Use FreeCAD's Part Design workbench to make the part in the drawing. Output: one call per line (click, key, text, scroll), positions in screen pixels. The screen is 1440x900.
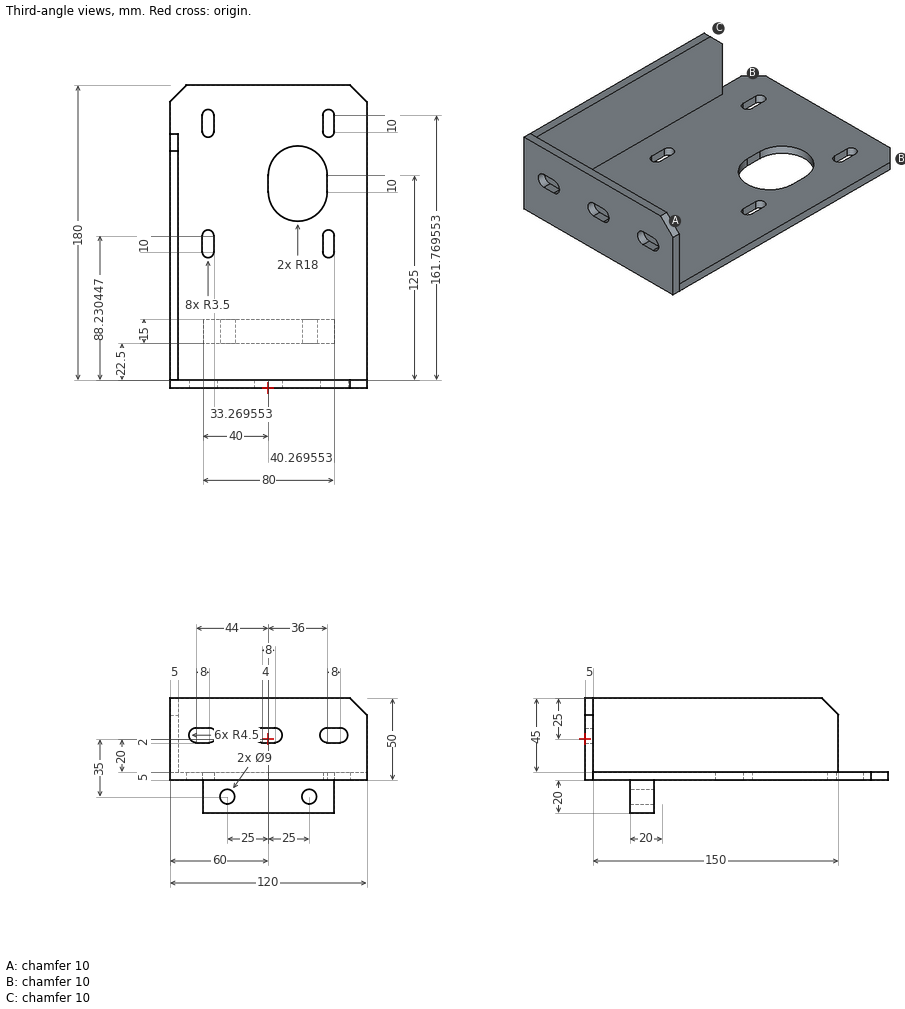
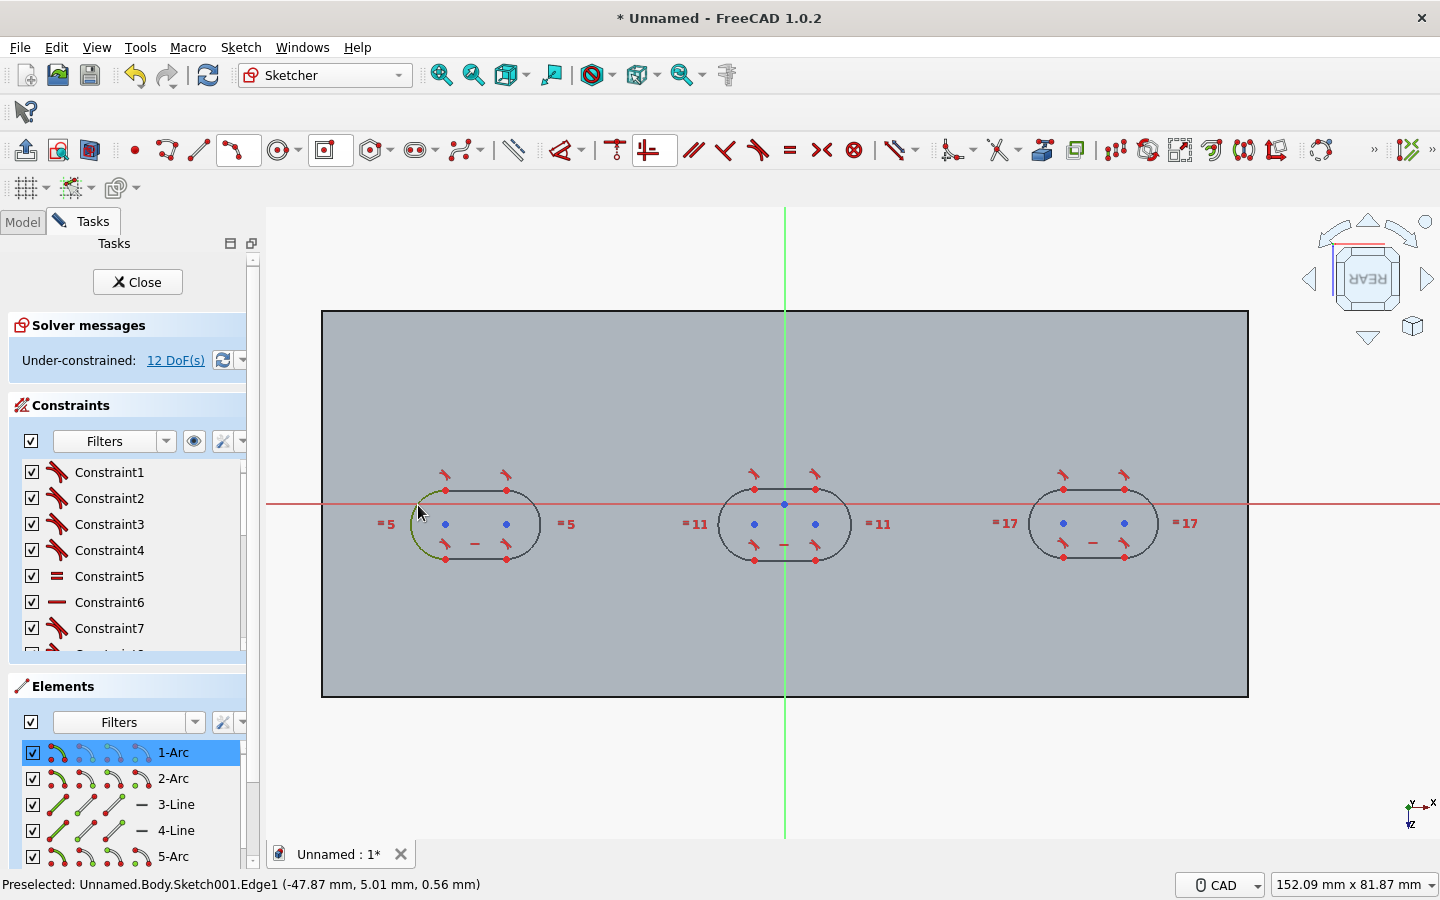
click(725, 504)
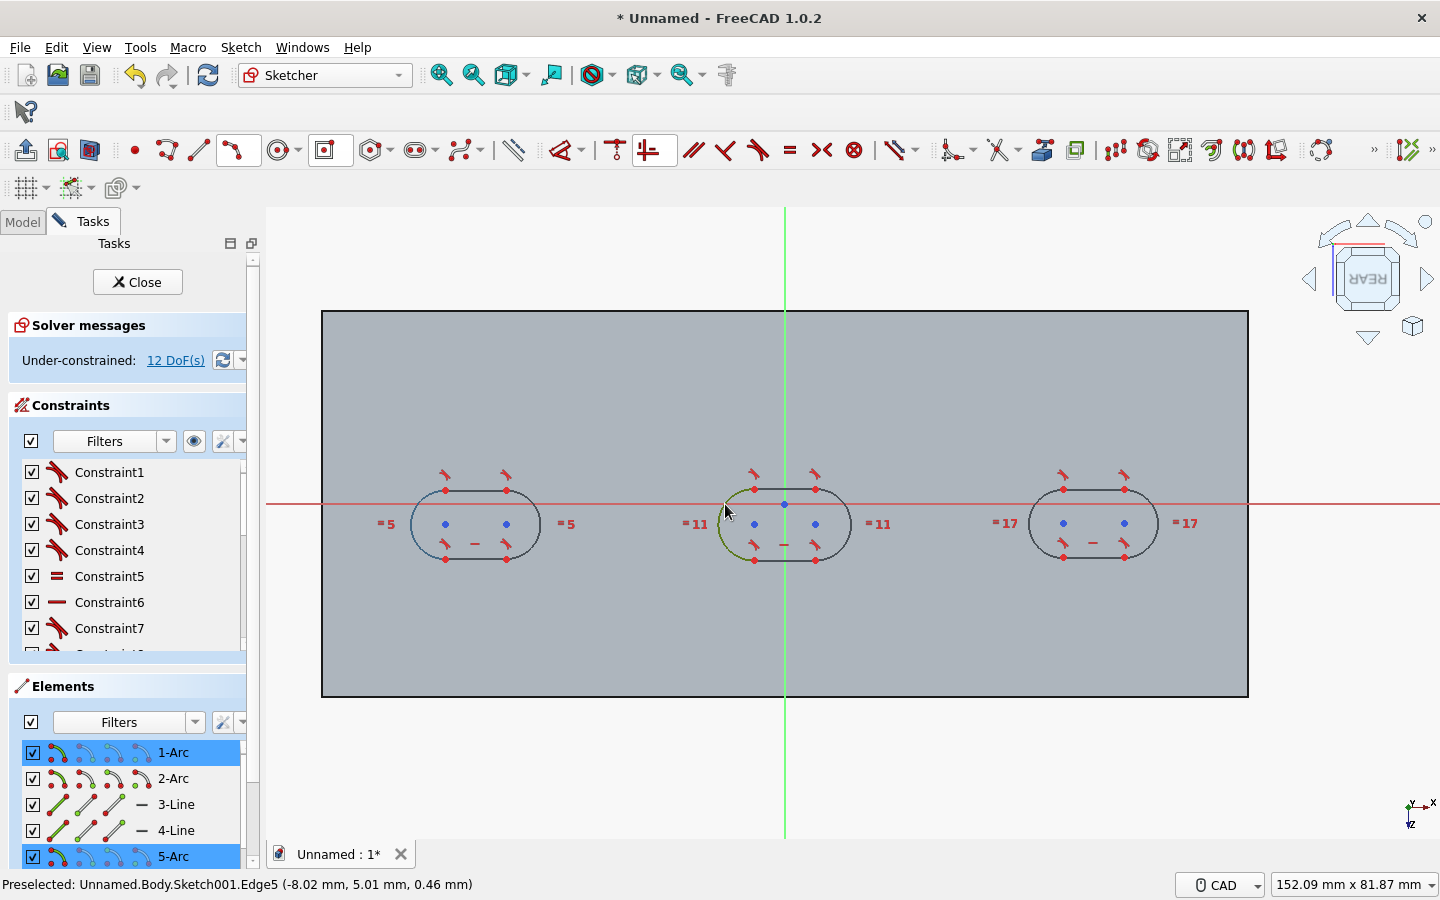
click(1035, 504)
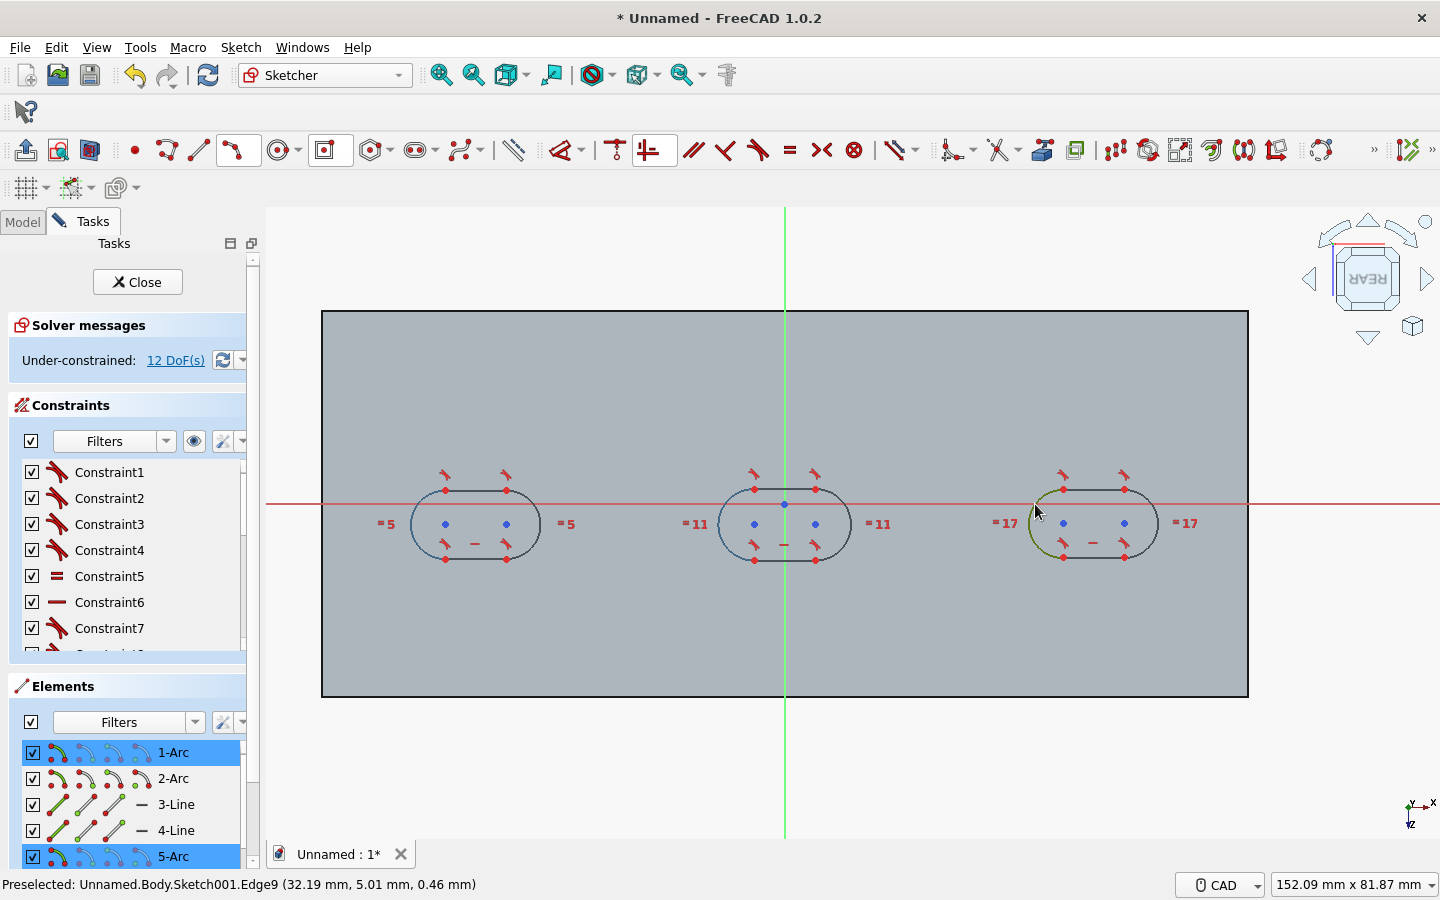
click(790, 150)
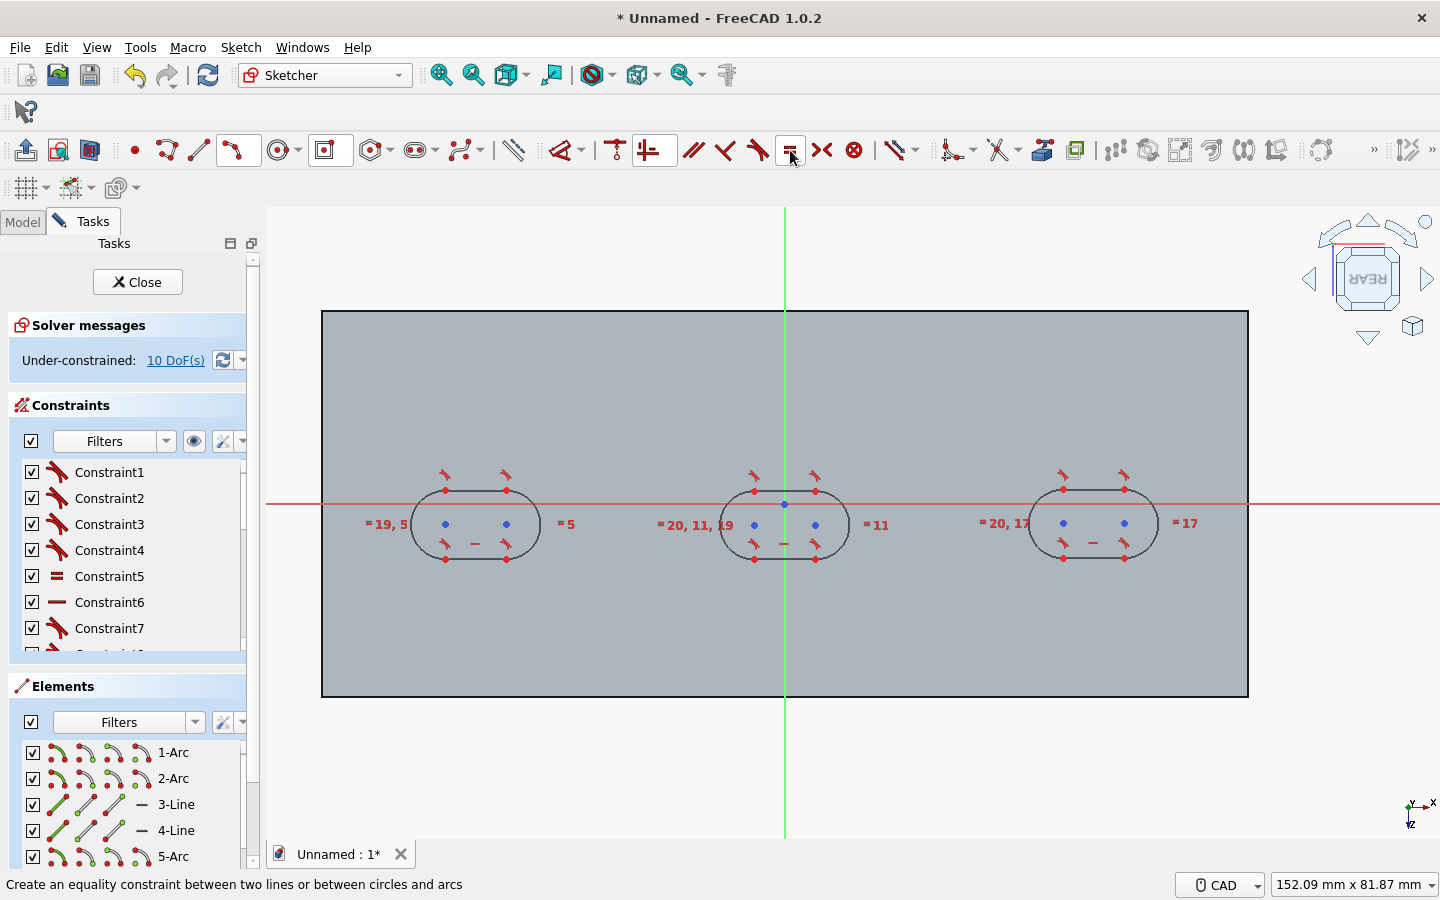
key(d)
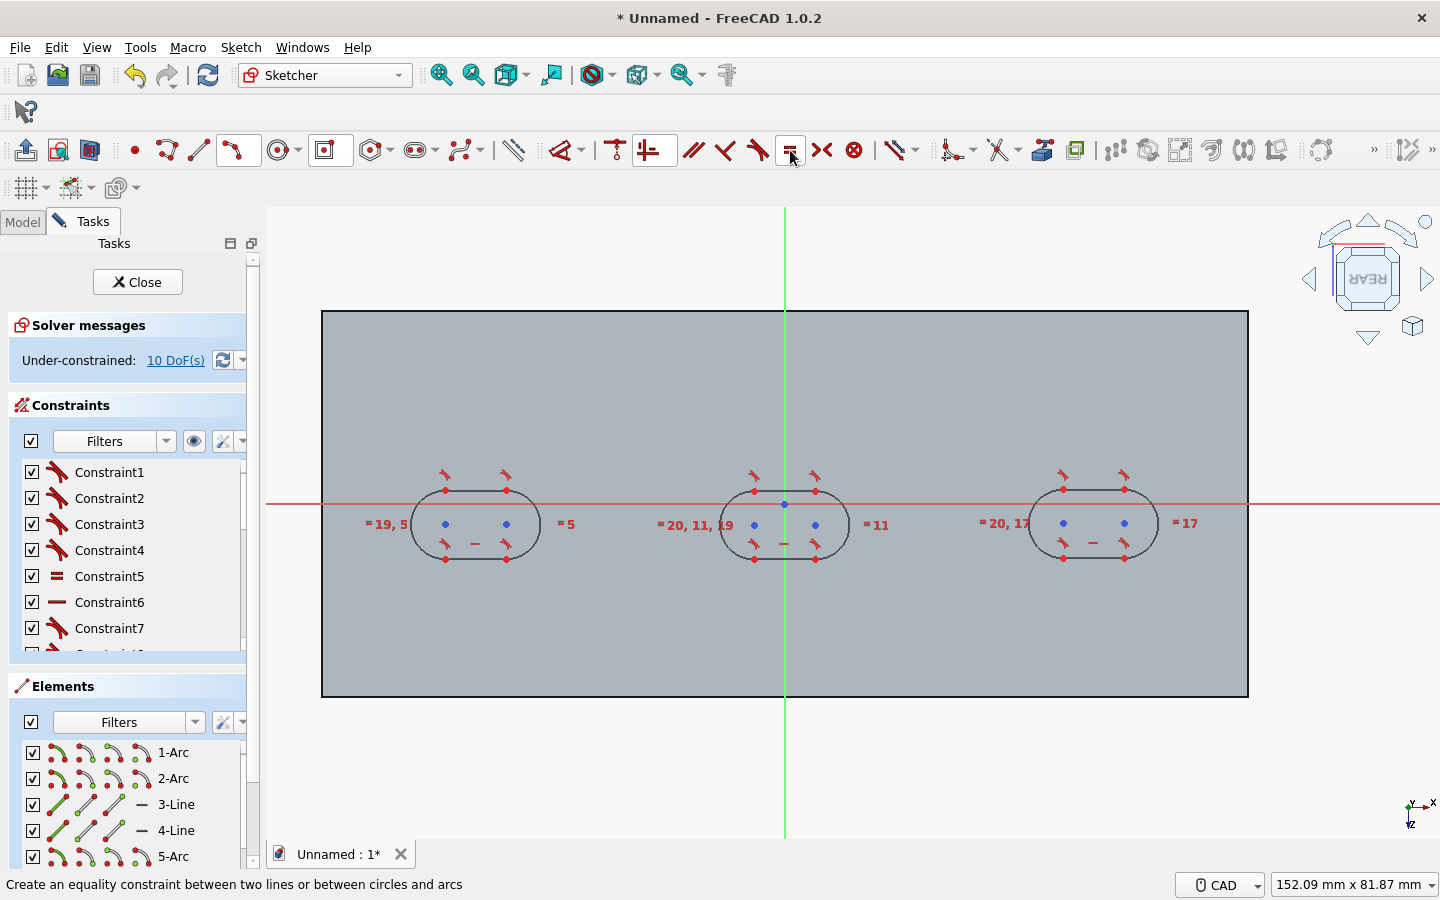
click(418, 505)
click(392, 486)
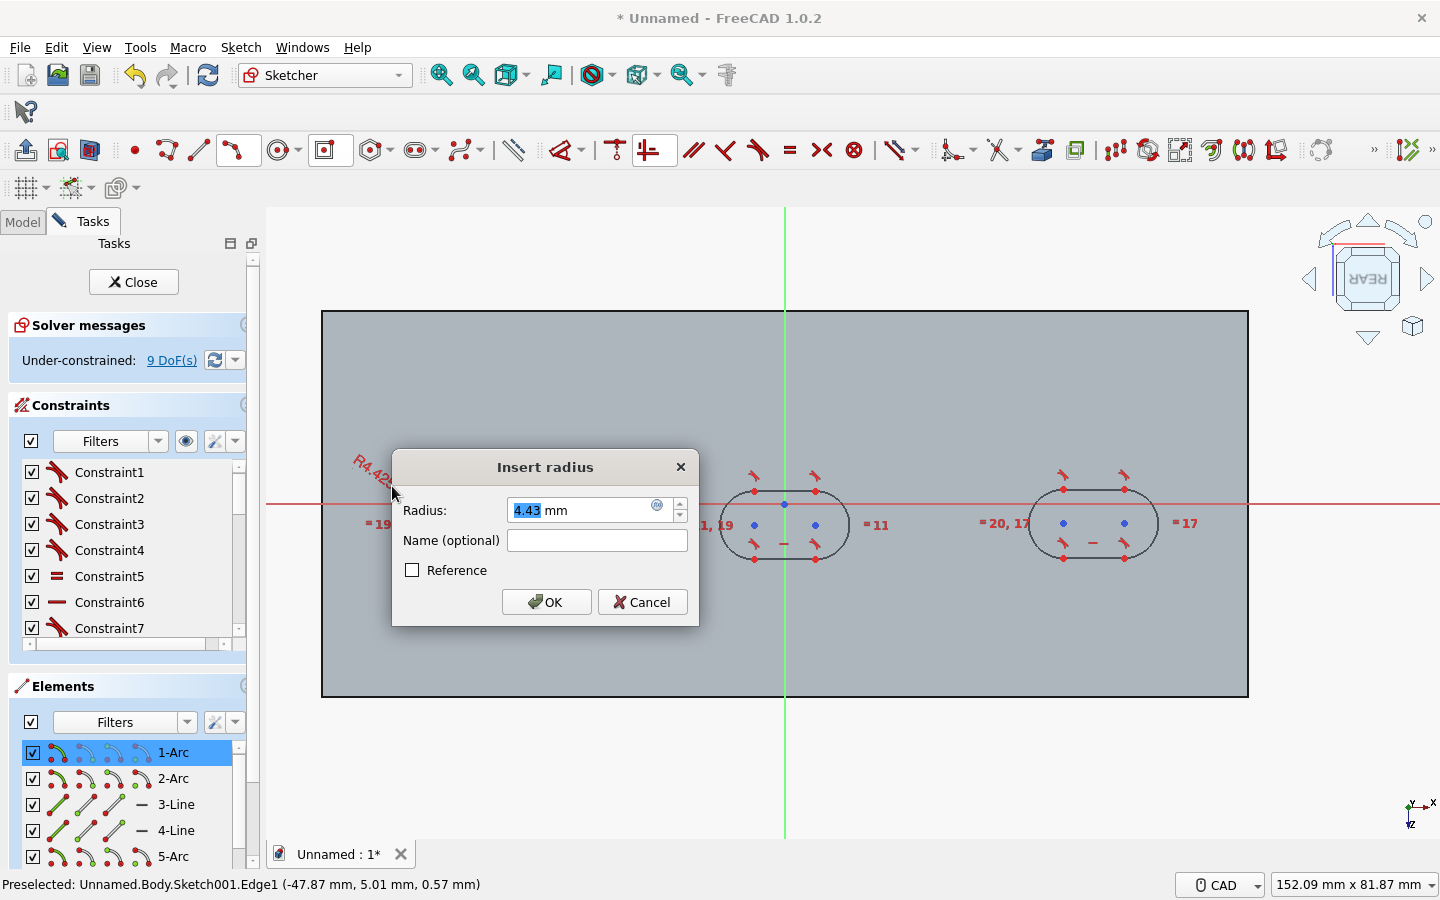
text(4.5)
key(Return)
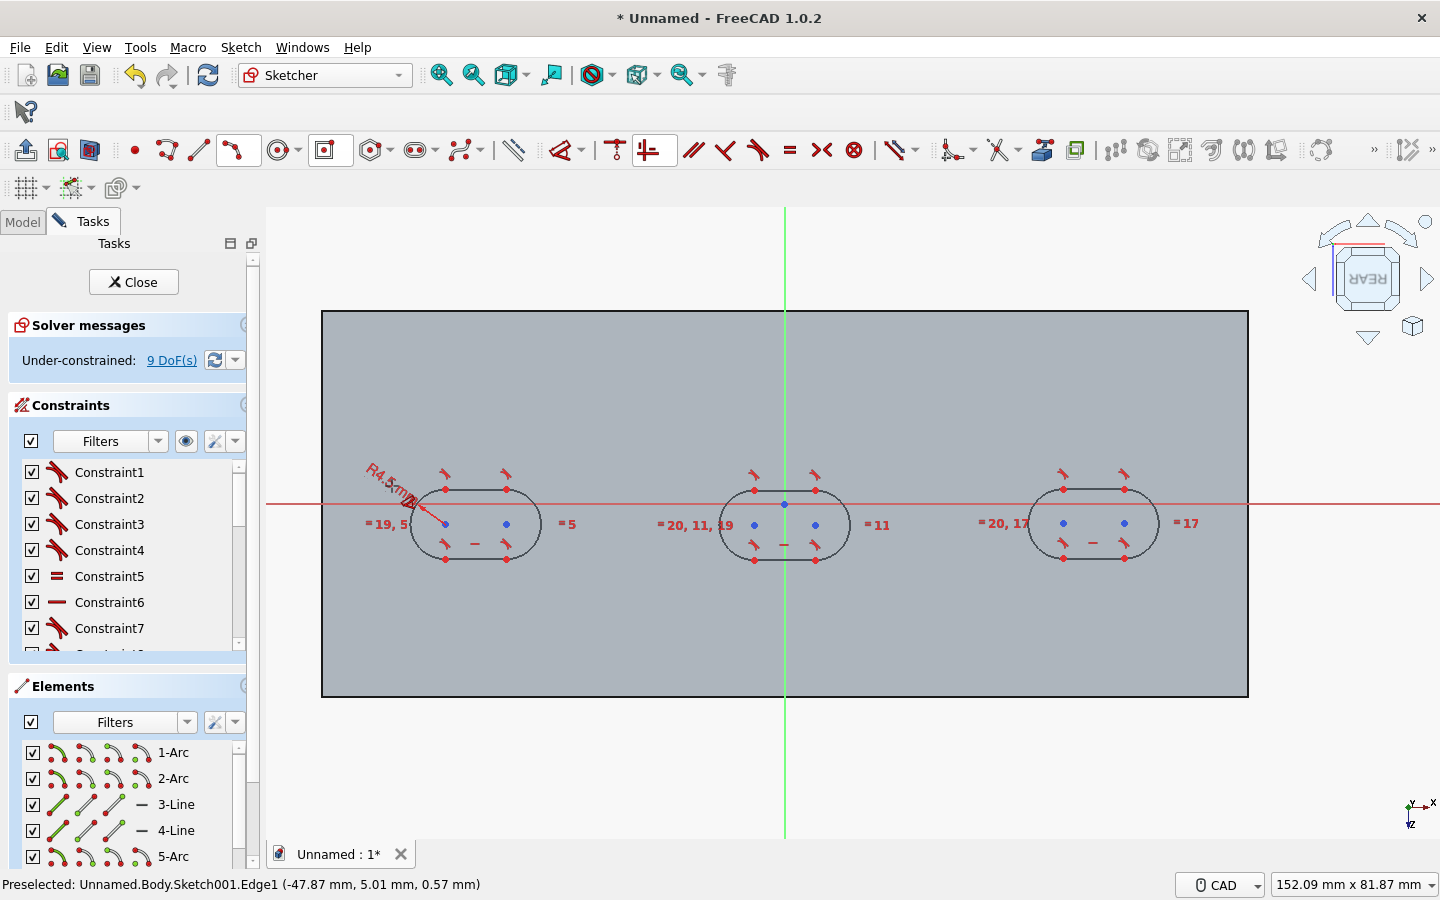
click(464, 490)
click(476, 456)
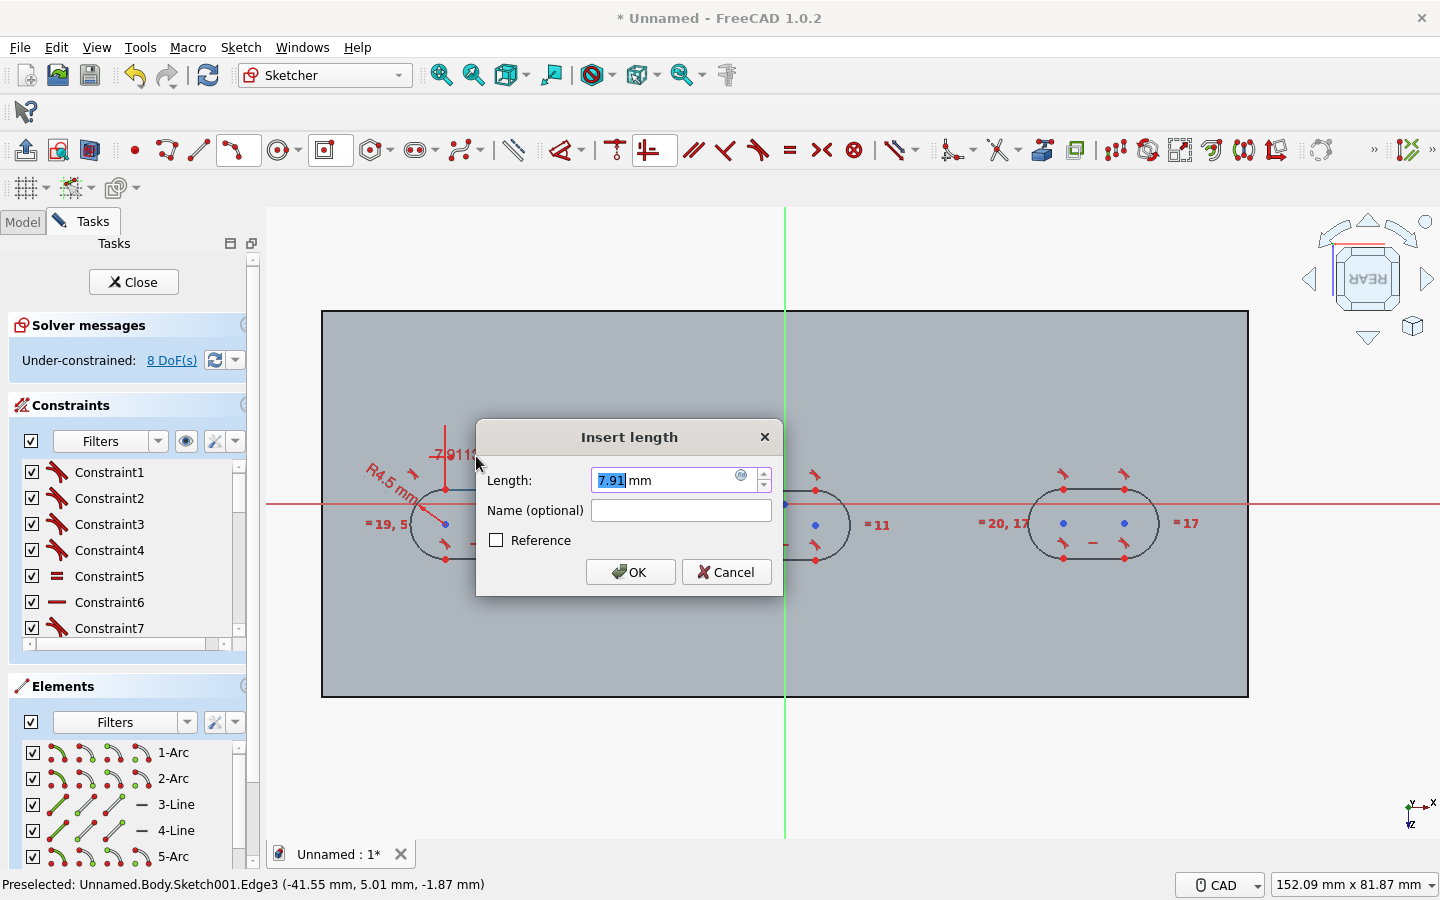
text(8)
key(Return)